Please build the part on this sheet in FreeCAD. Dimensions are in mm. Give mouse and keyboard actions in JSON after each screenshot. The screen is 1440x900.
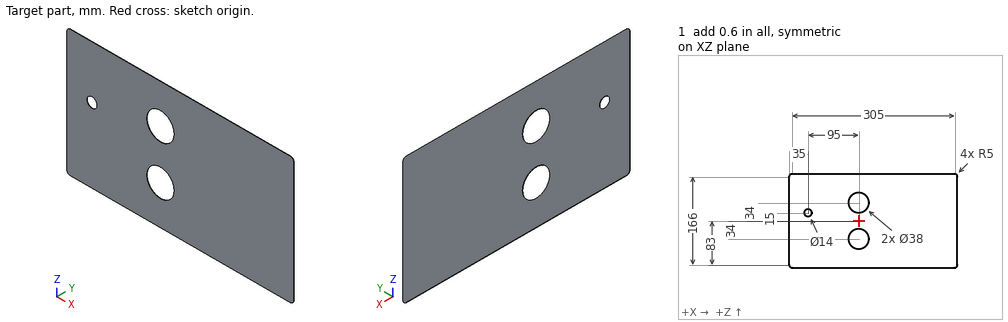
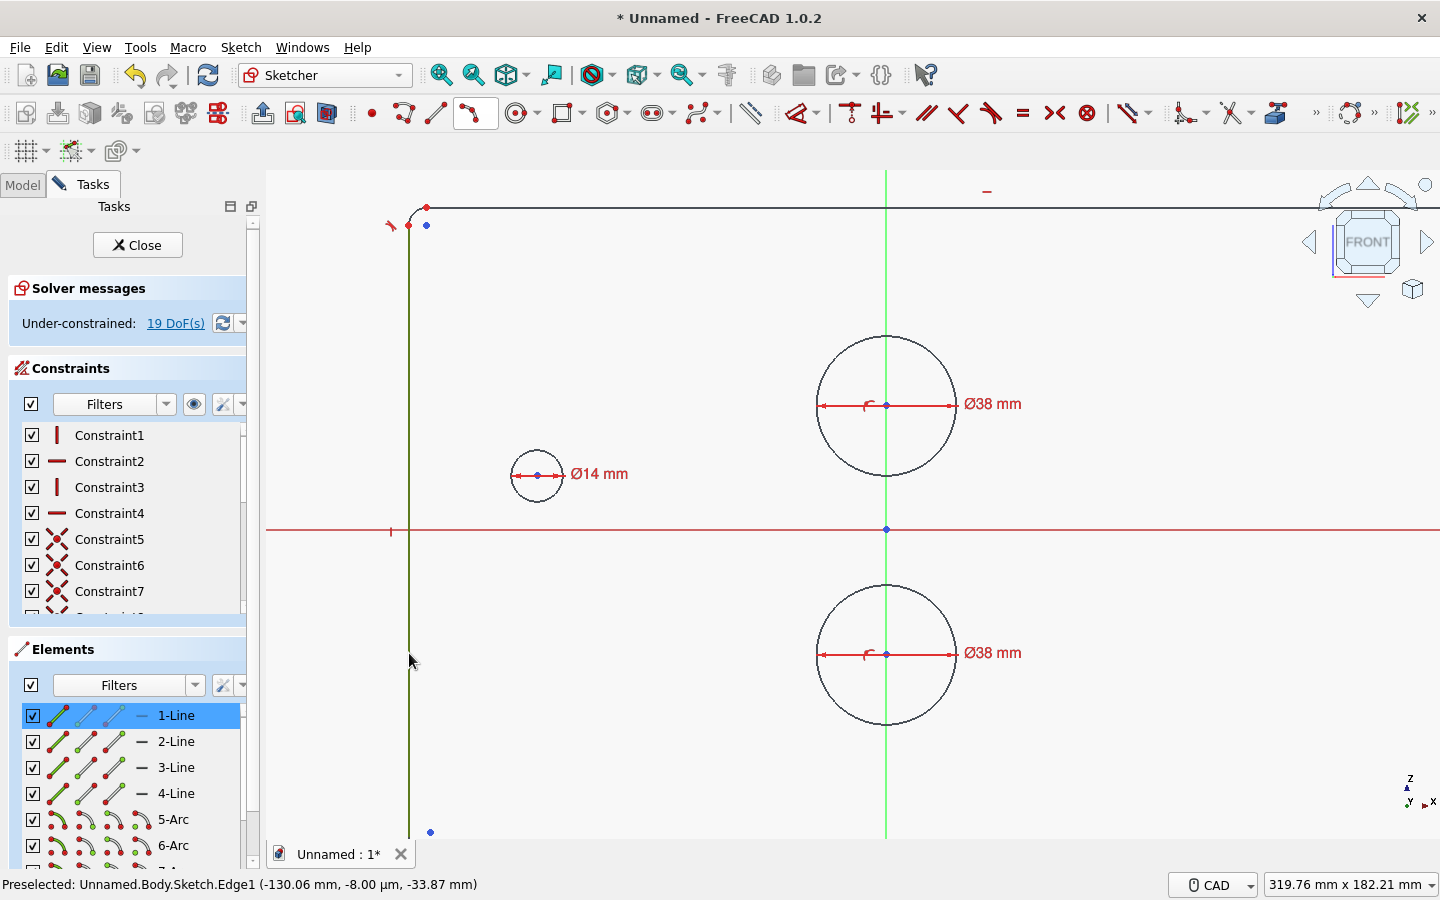
{"action": "scroll", "coordinate": [538, 474], "scroll_direction": "down", "scroll_amount": 3}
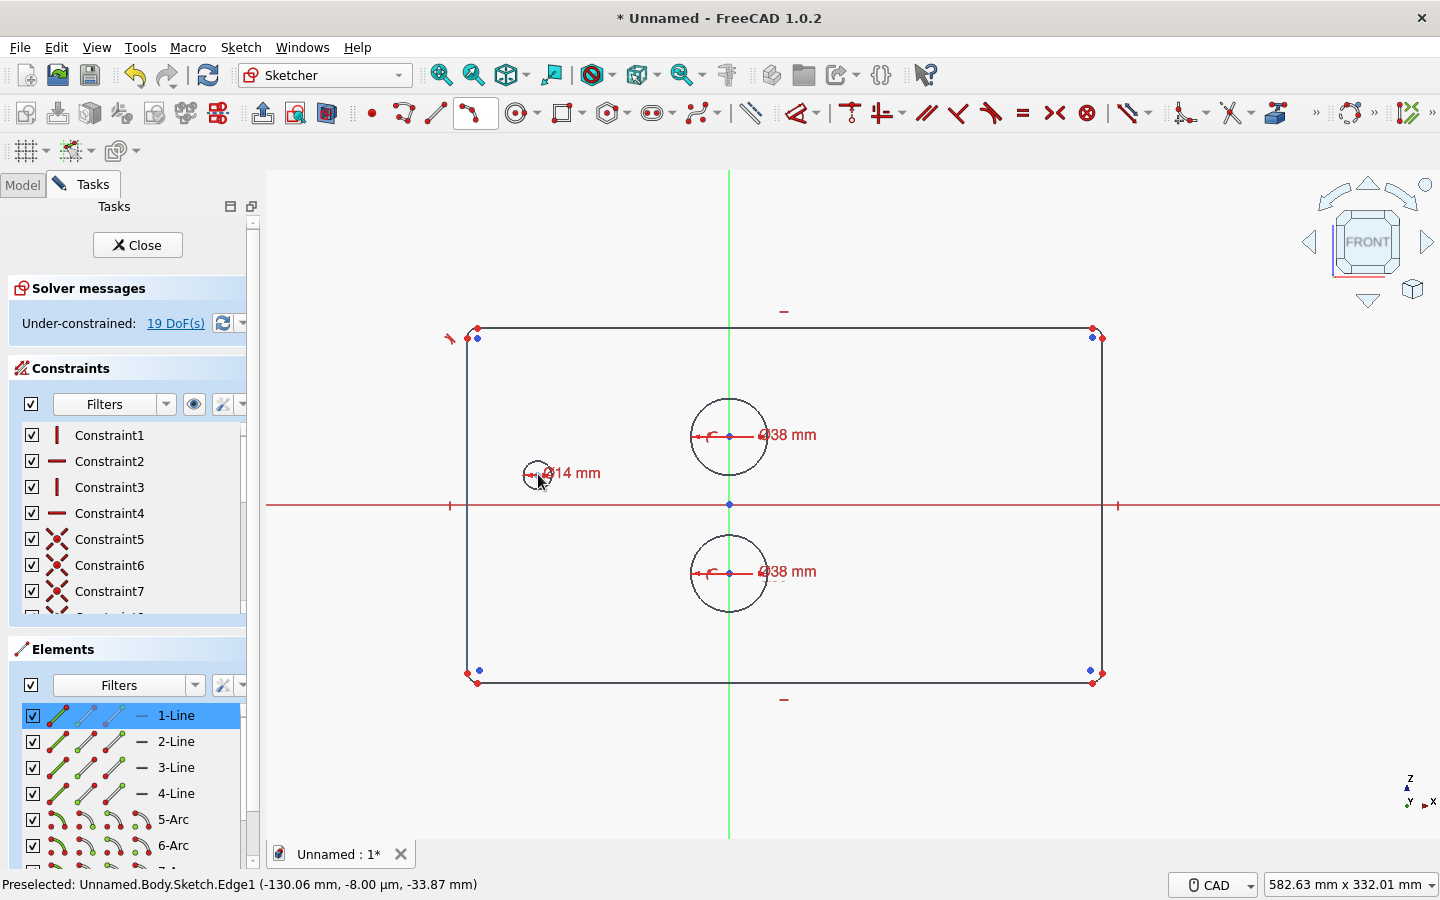
{"action": "scroll", "coordinate": [471, 680], "scroll_direction": "up", "scroll_amount": 4}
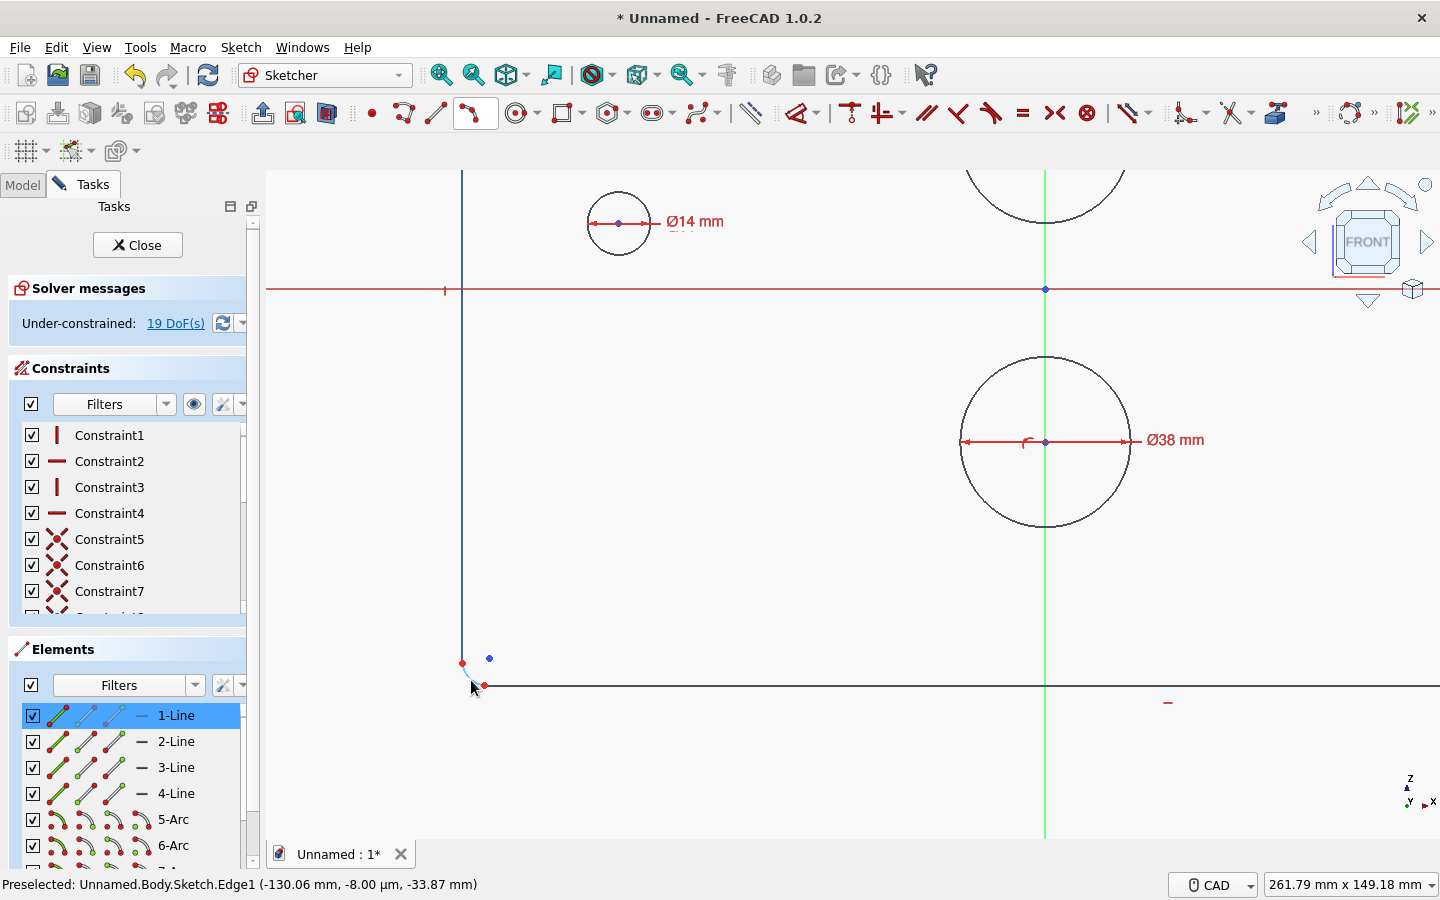
{"action": "left_click", "coordinate": [470, 678]}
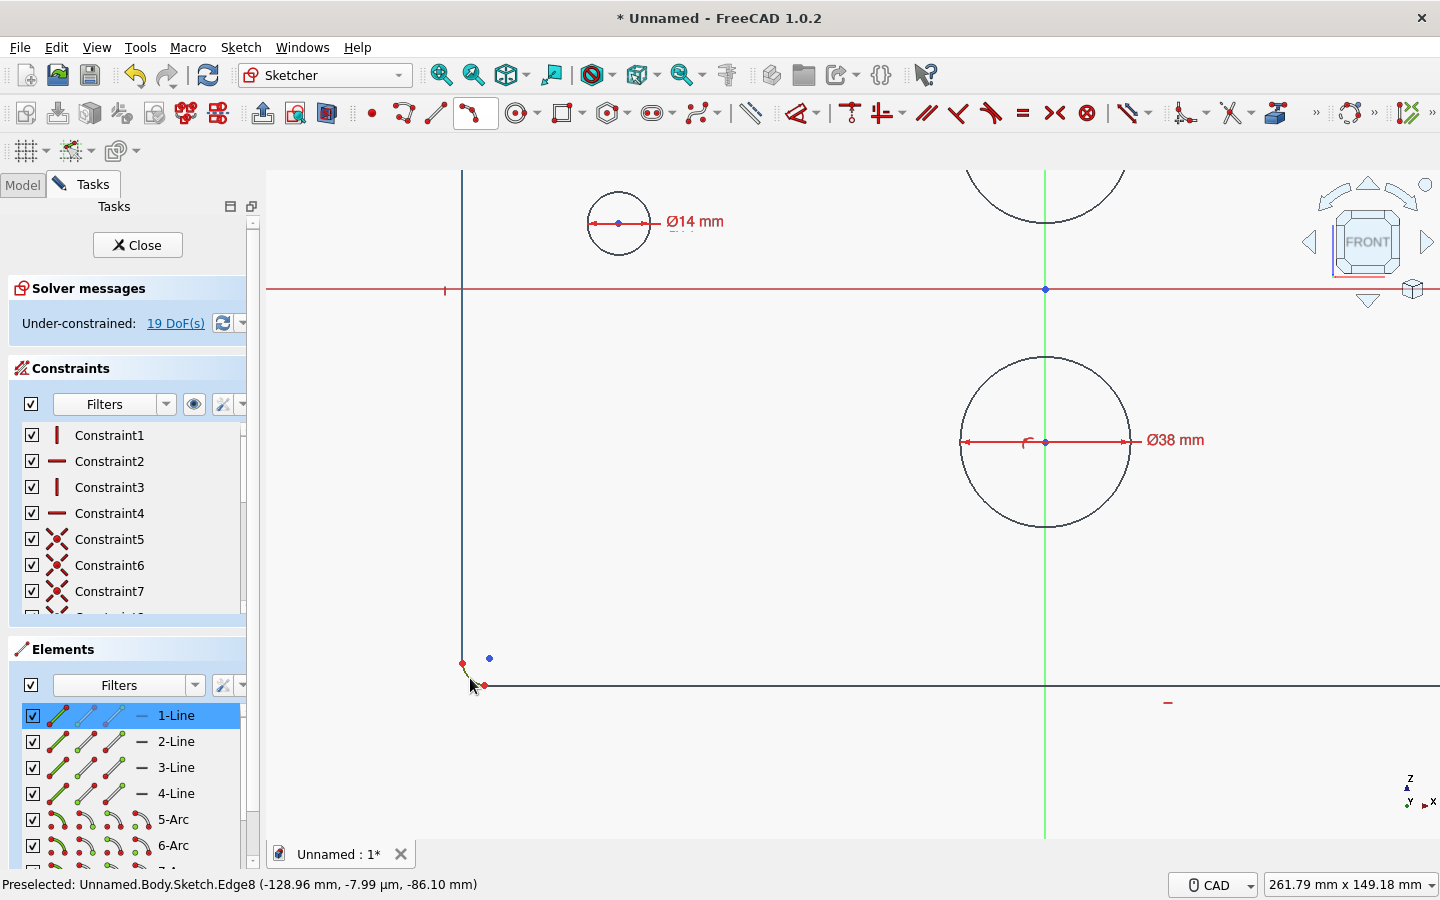
{"action": "left_click", "coordinate": [992, 114]}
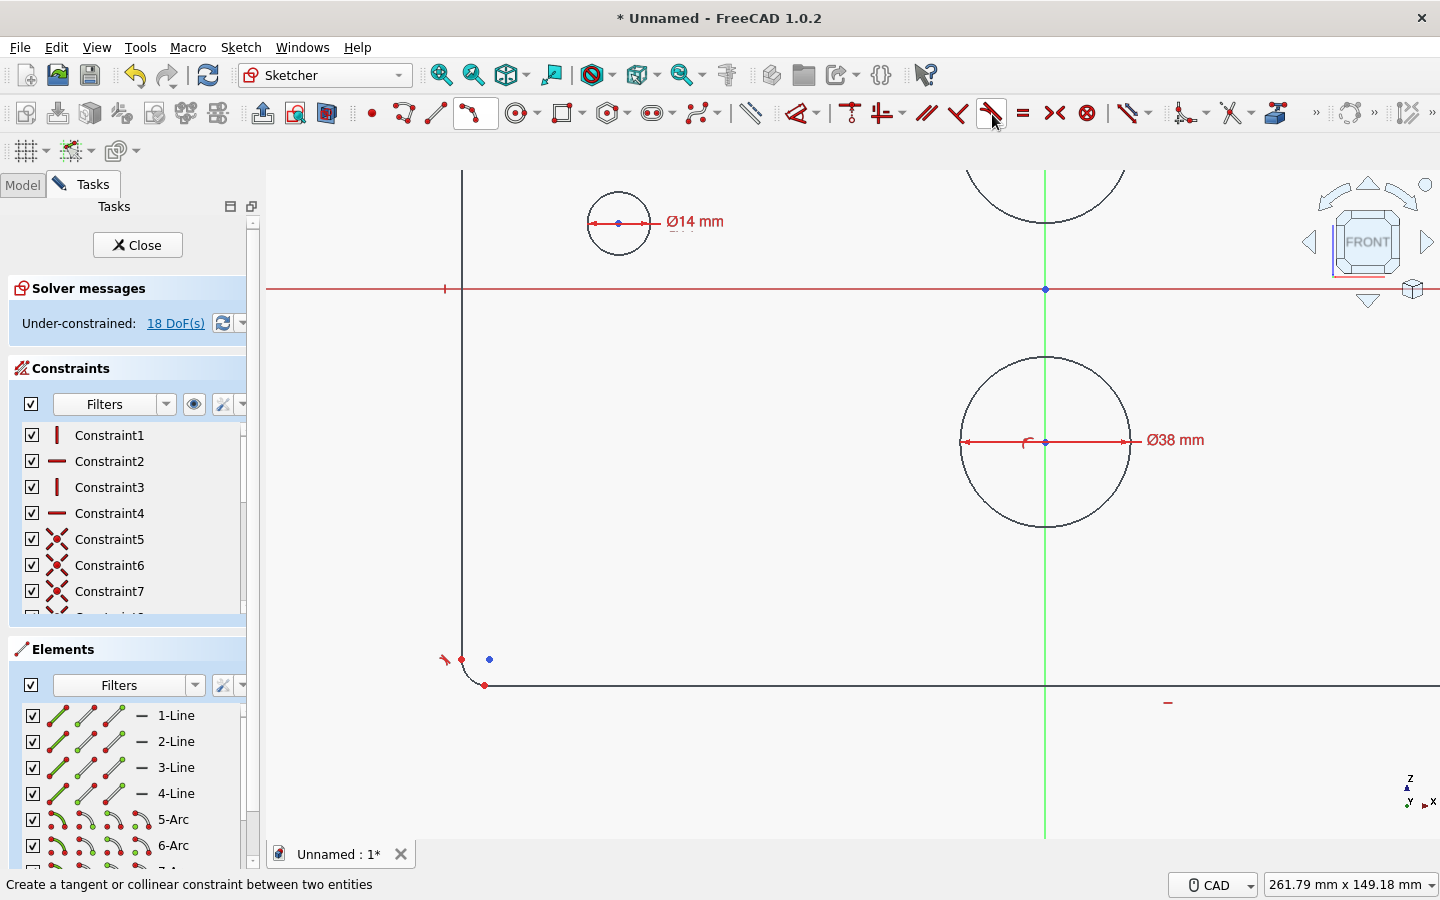
{"action": "scroll", "coordinate": [471, 680], "scroll_direction": "down", "scroll_amount": 4}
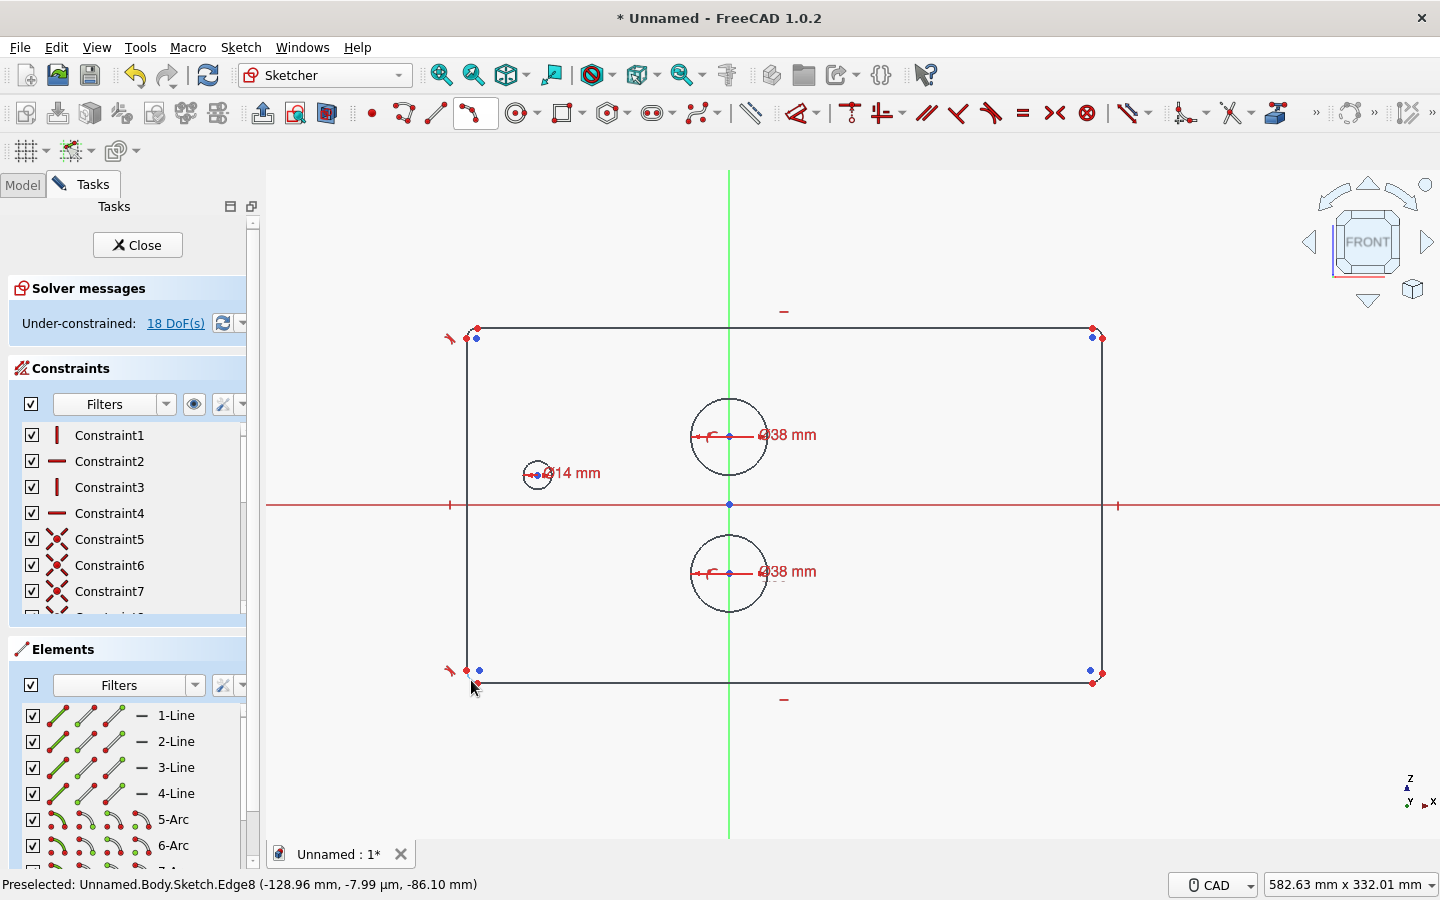
{"action": "left_click", "coordinate": [662, 328]}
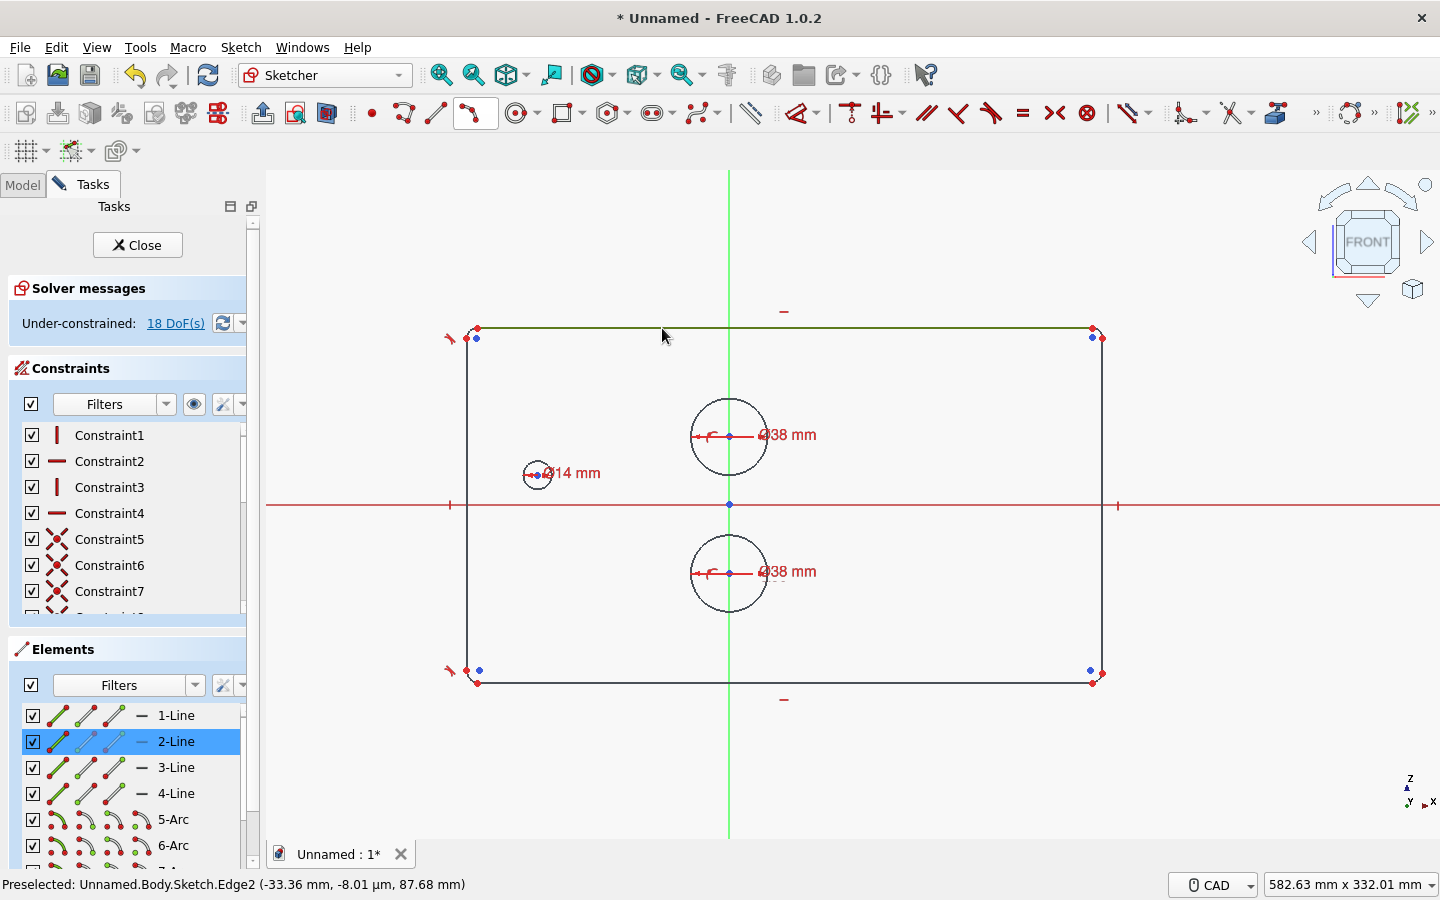
{"action": "scroll", "coordinate": [470, 331], "scroll_direction": "up", "scroll_amount": 3}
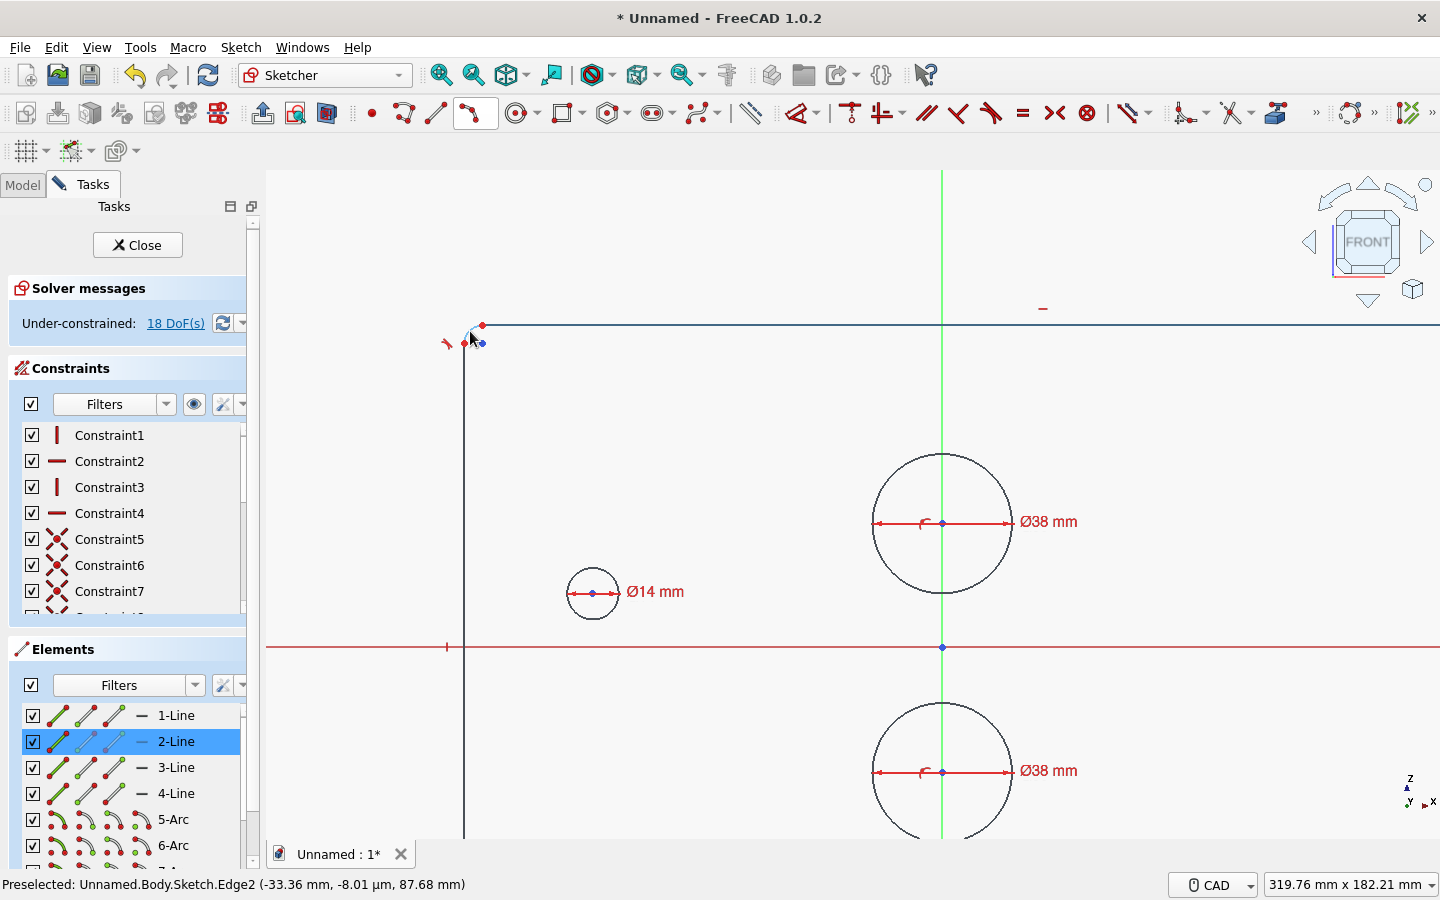
{"action": "left_click", "coordinate": [470, 331]}